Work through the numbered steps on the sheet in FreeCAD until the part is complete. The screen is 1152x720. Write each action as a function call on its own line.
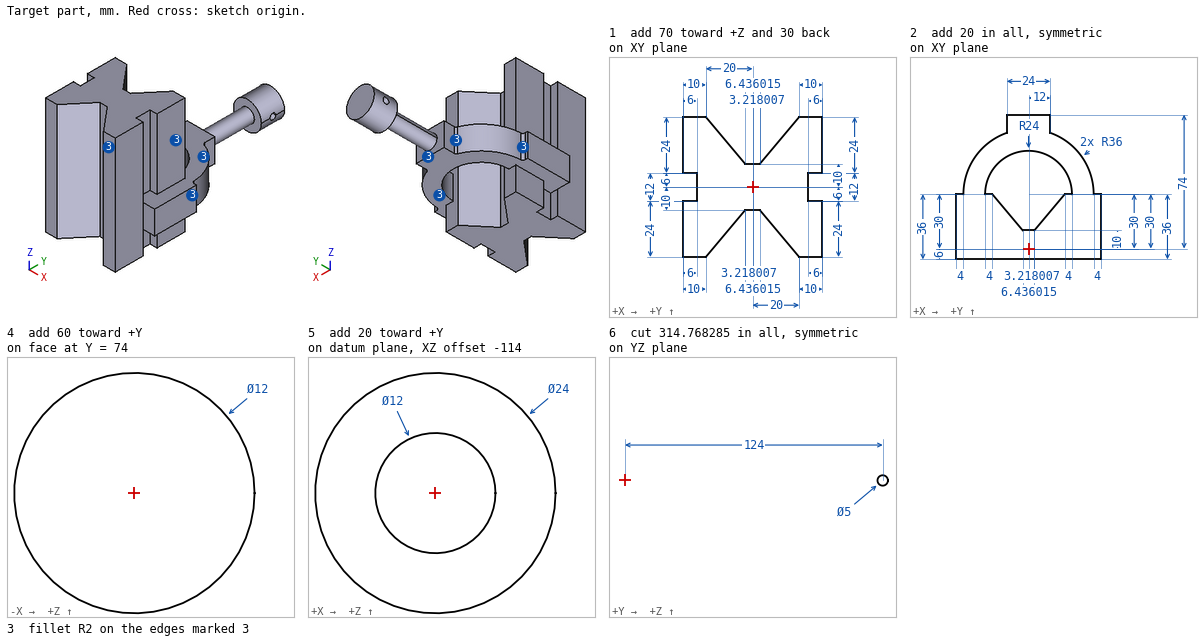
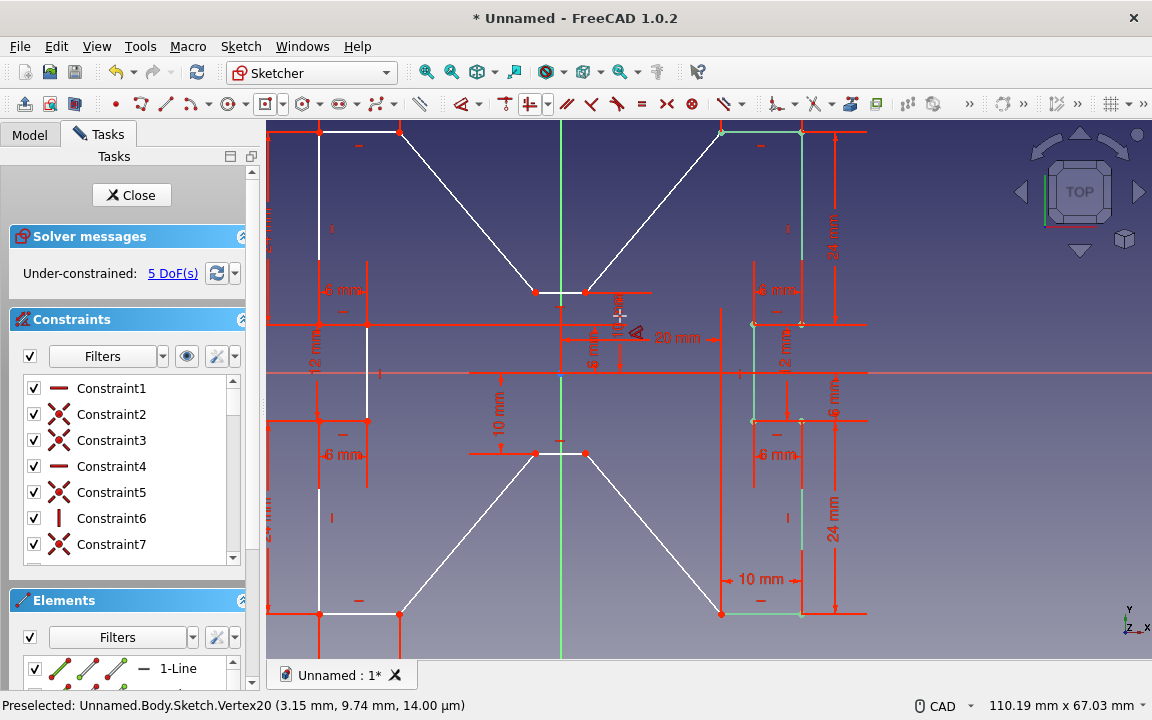
scroll(803, 423, down, 2)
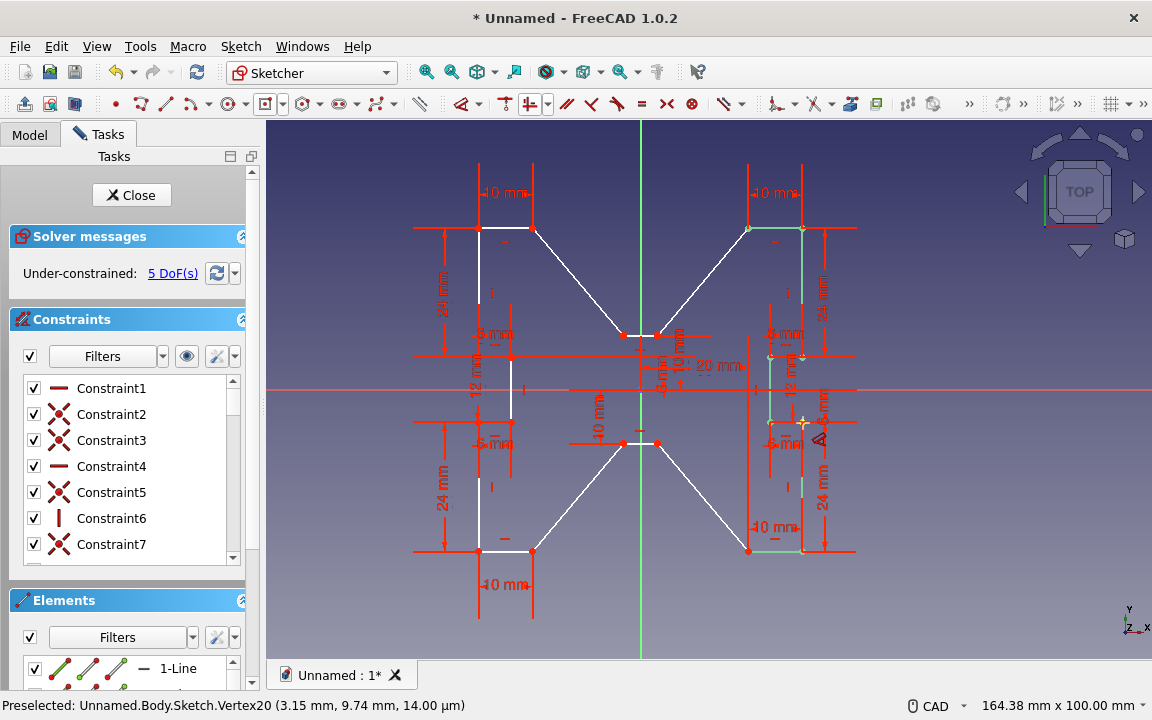
click(533, 228)
click(587, 194)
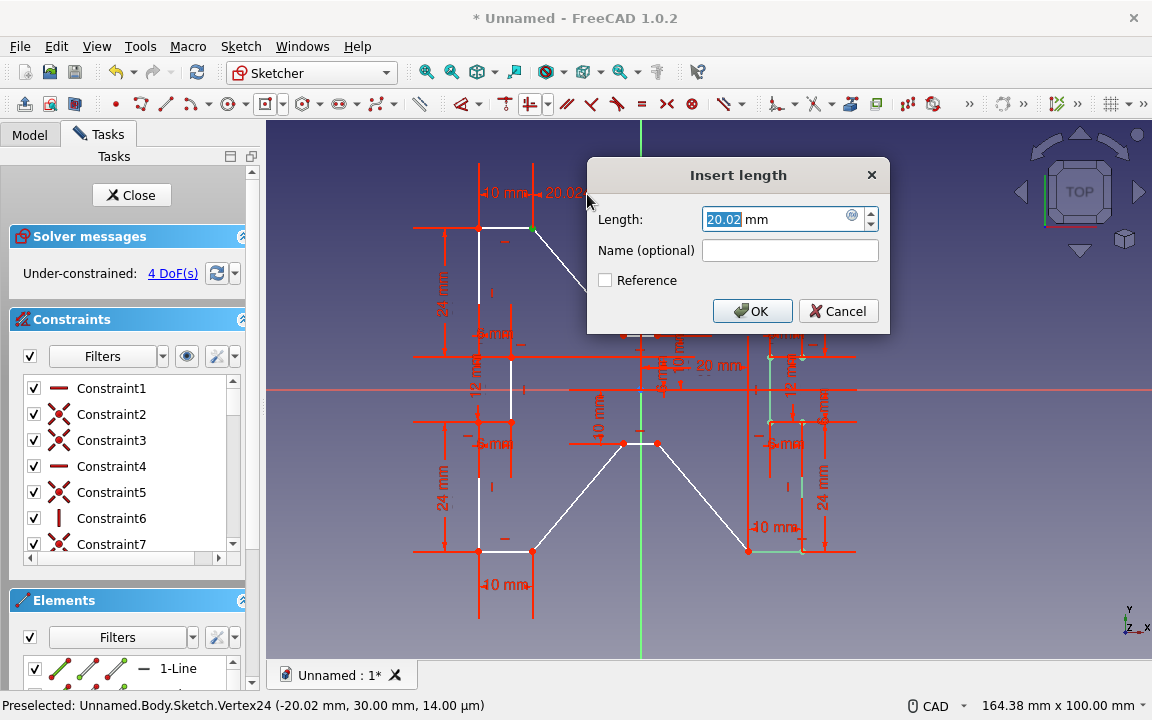
text(20)
key(Return)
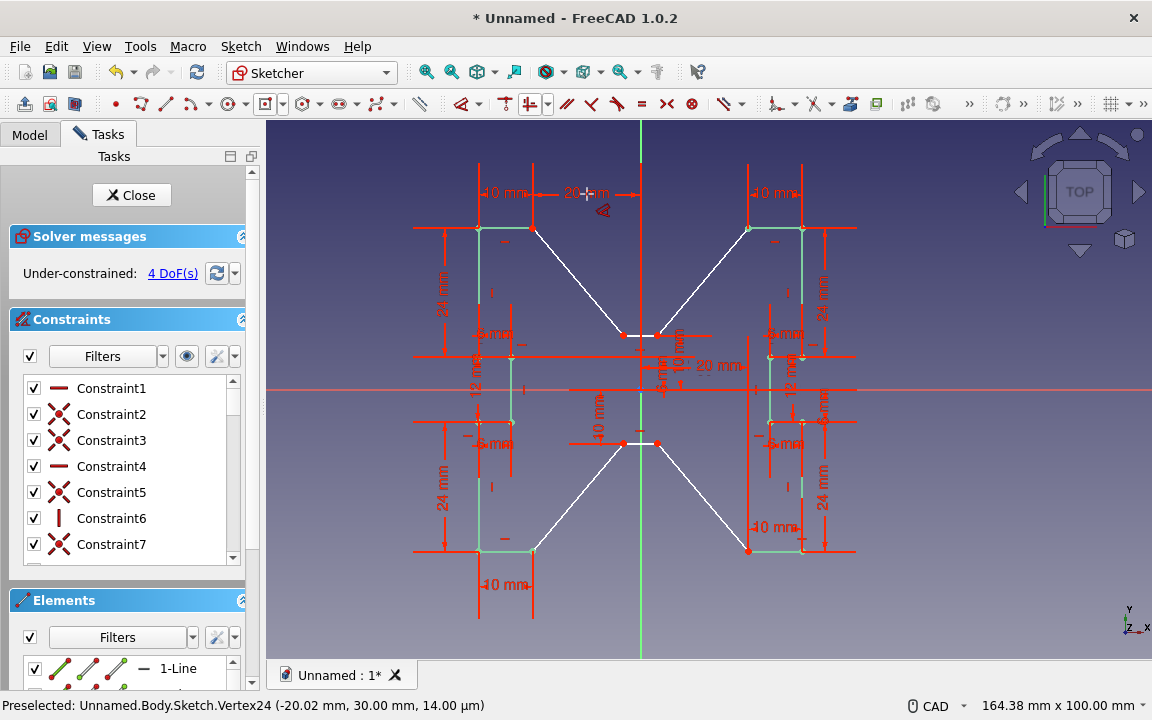
click(637, 444)
click(633, 478)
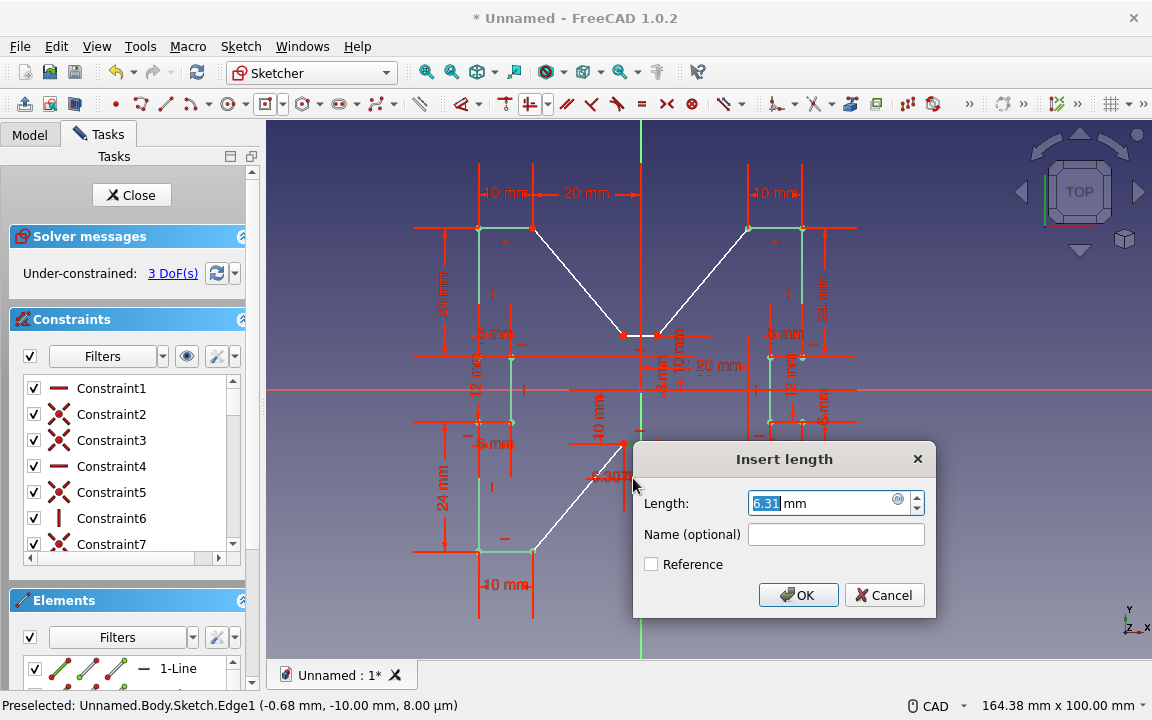
text(6.436015)
key(Return)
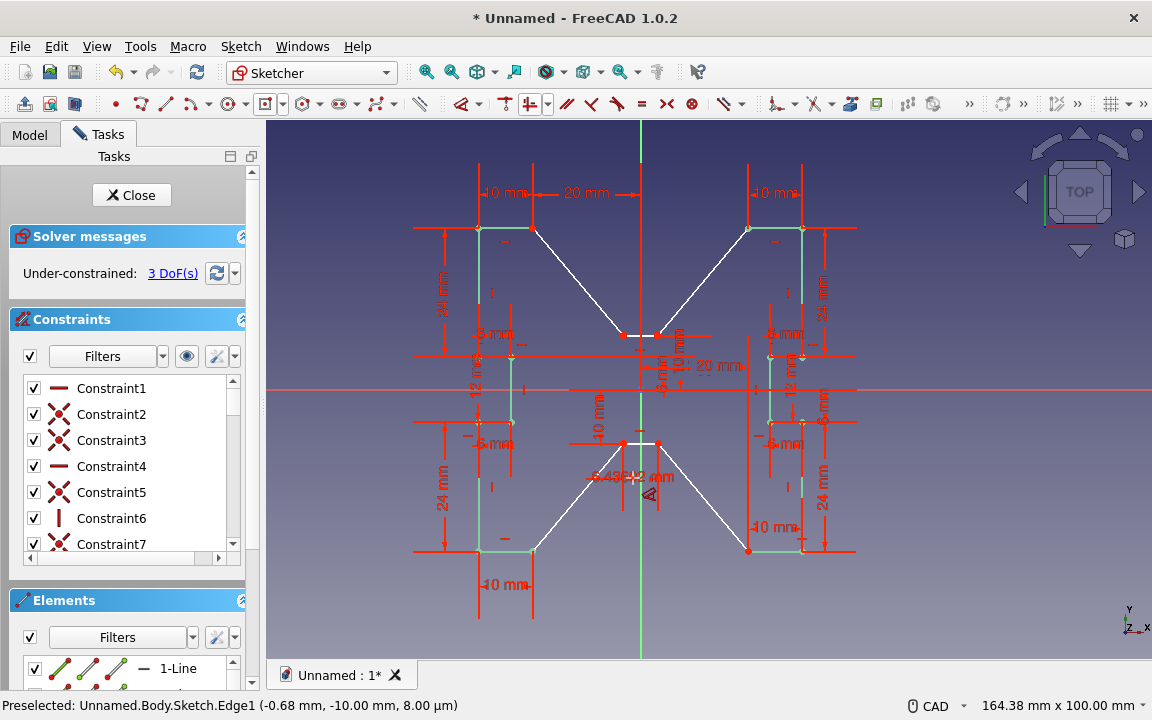
click(644, 336)
click(633, 302)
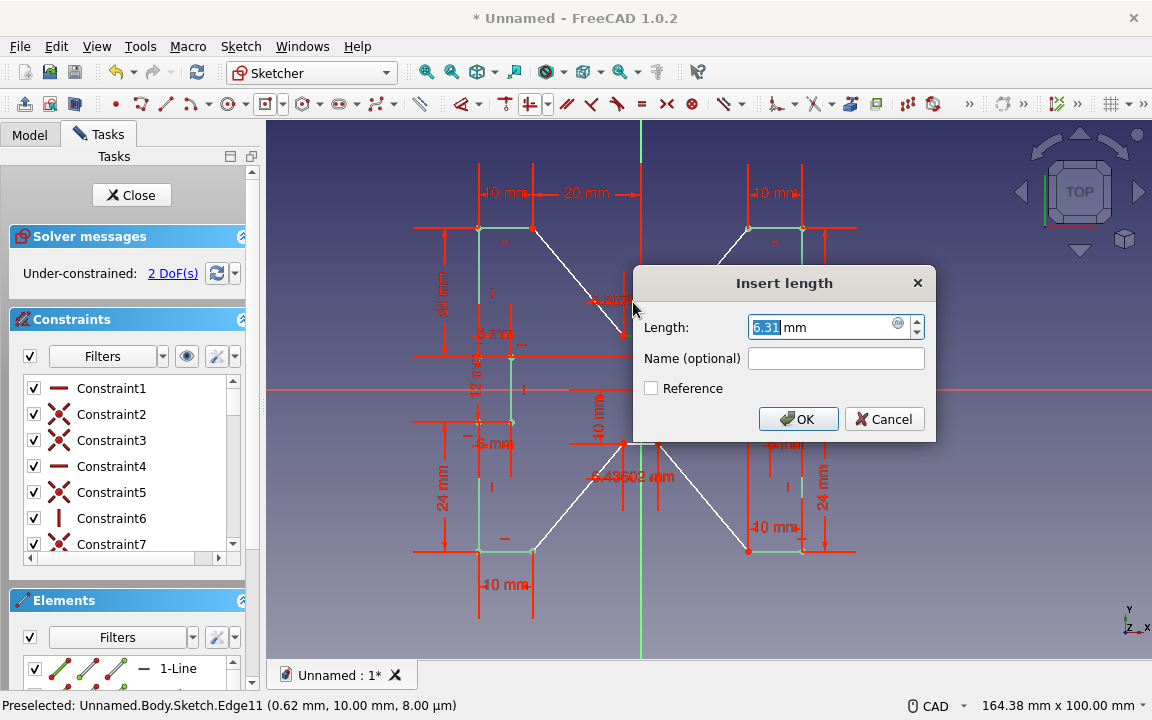
text(6.436015)
key(Return)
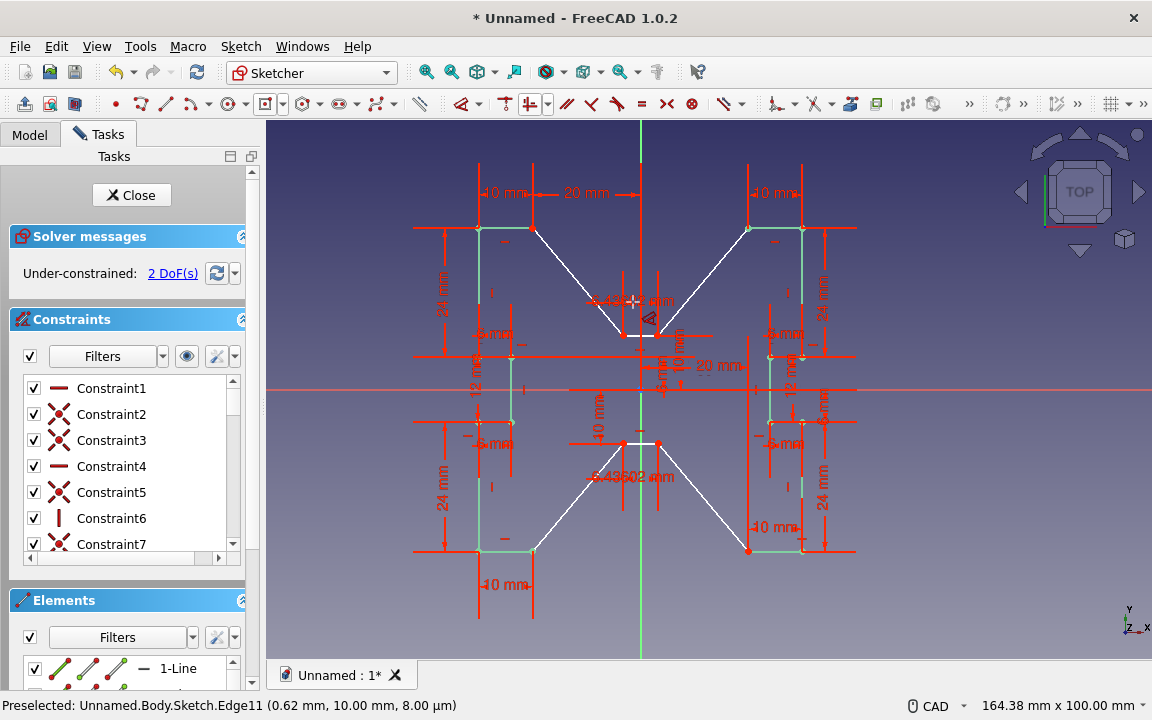
scroll(623, 444, up, 5)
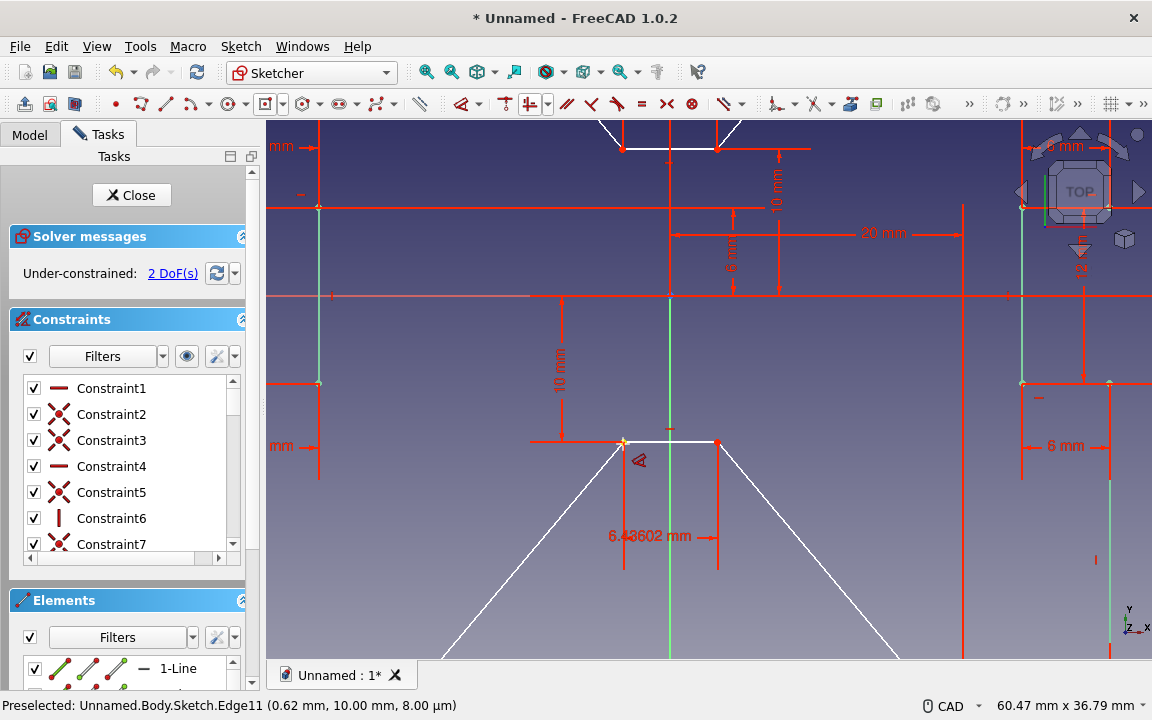
click(624, 442)
click(647, 476)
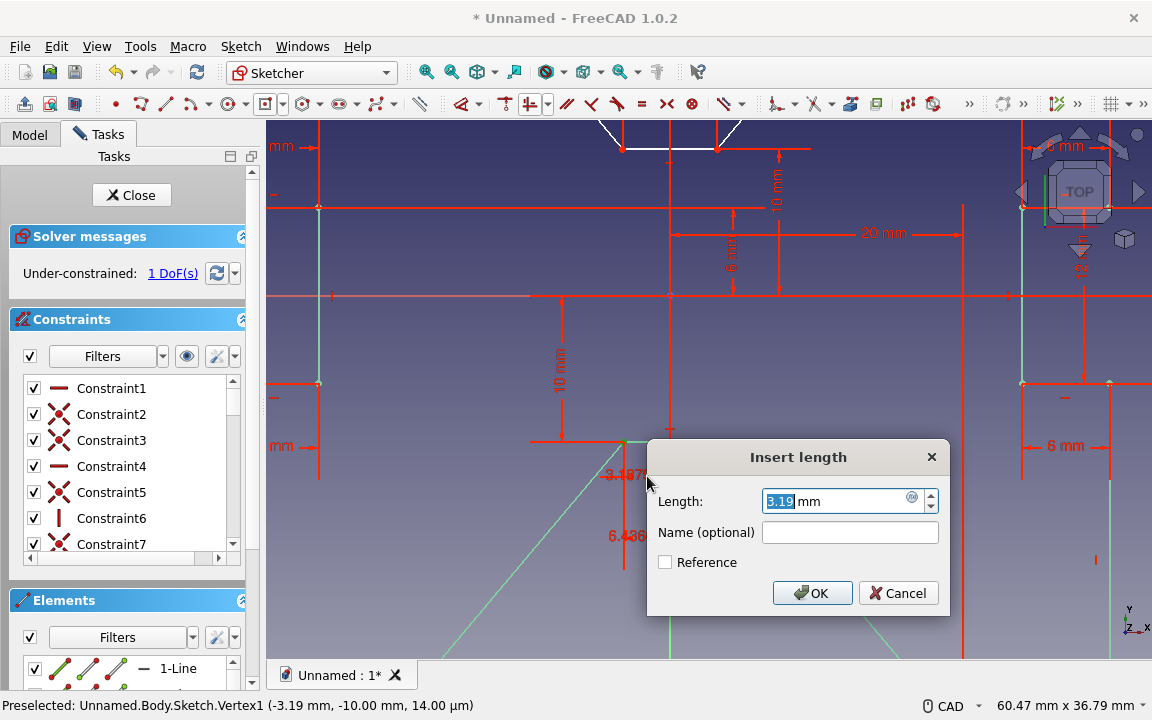
text(3.218007)
key(Return)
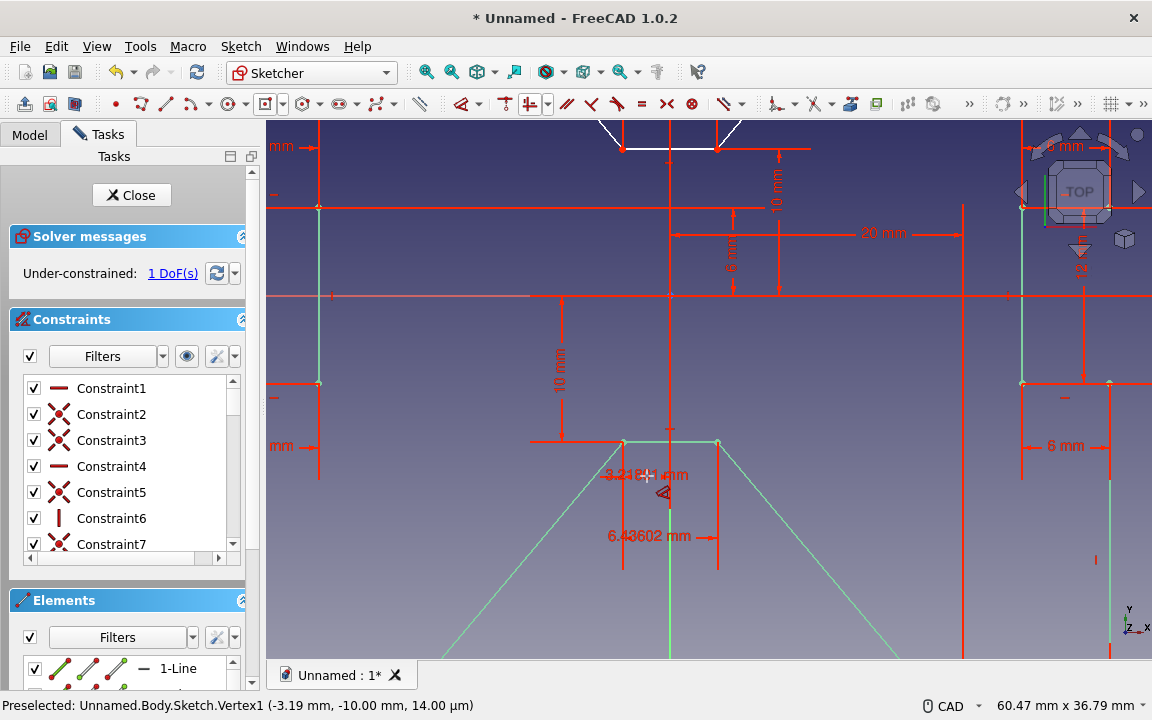
click(717, 149)
click(694, 330)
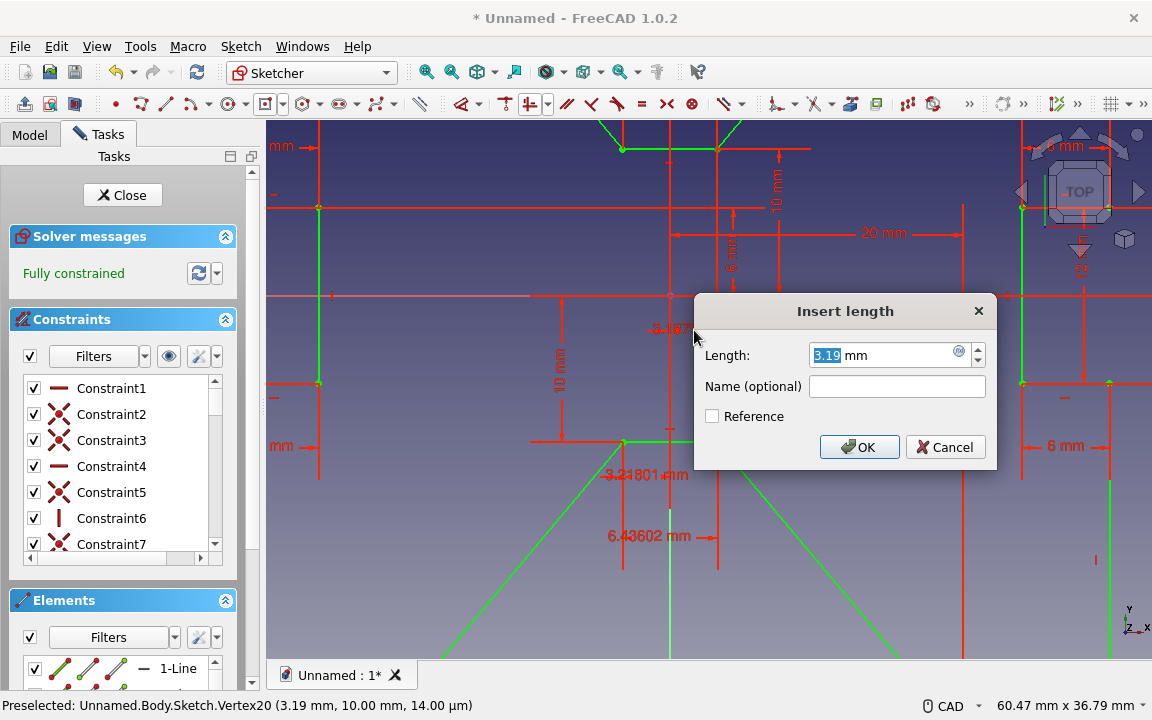
text(3.218007)
key(Return)
key(Escape)